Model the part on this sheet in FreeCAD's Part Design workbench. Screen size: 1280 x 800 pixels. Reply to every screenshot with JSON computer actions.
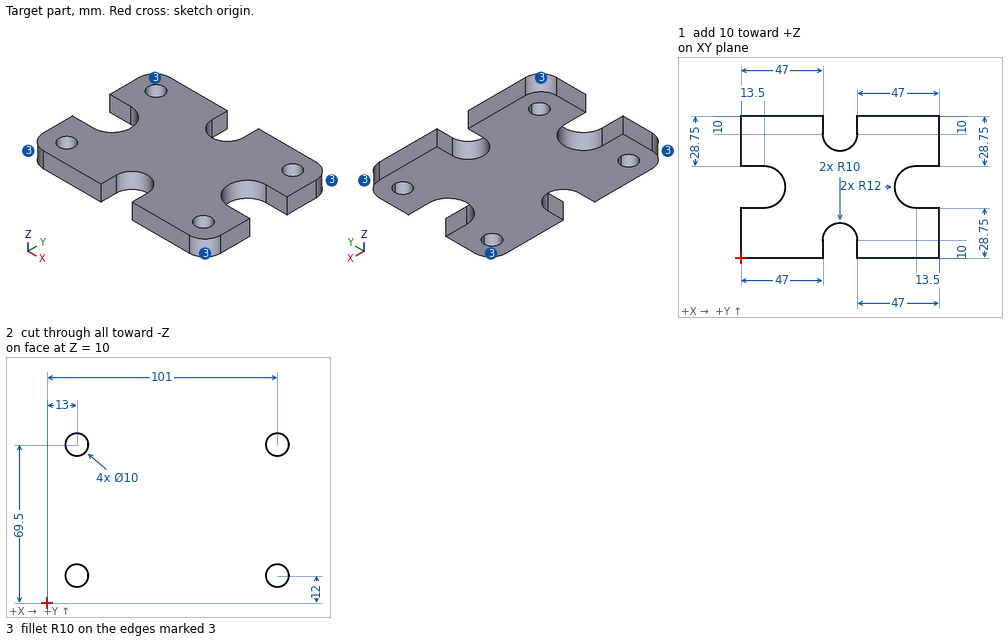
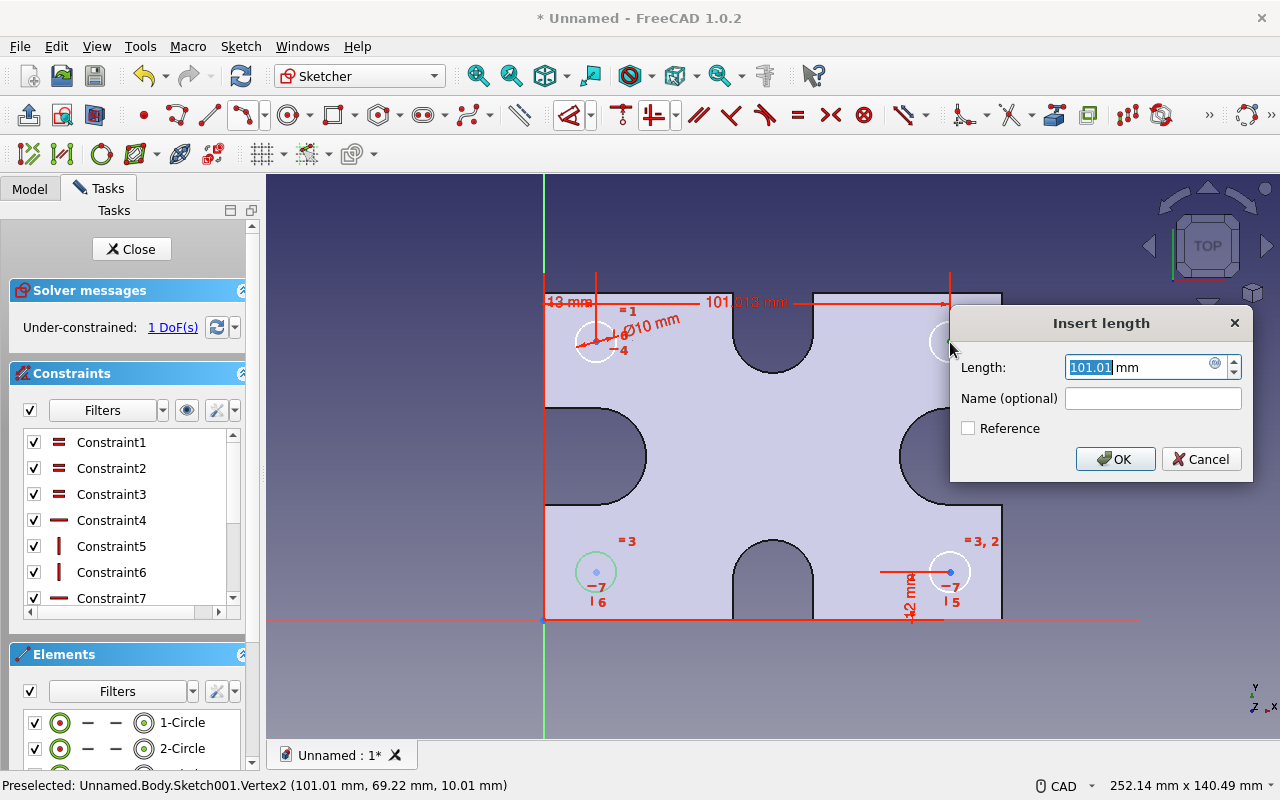
{"action": "type", "text": "101"}
{"action": "key", "text": "Return"}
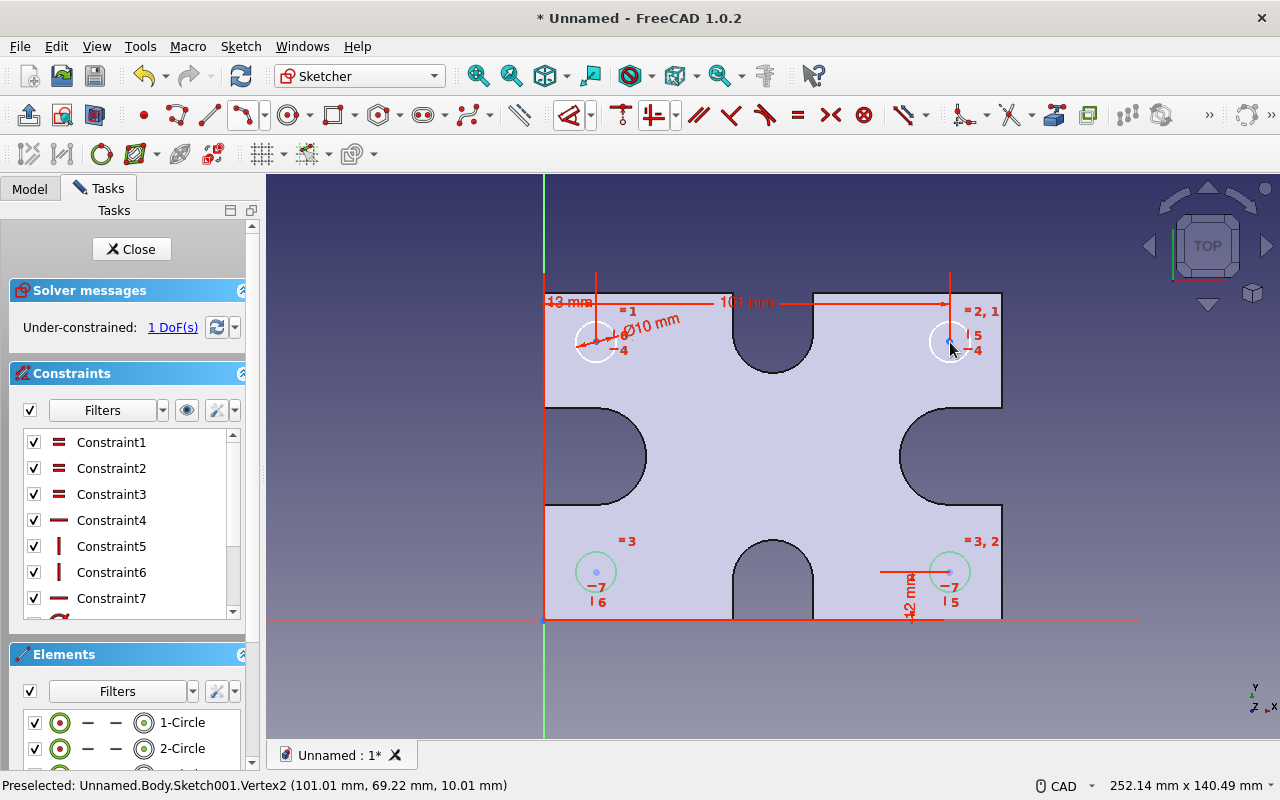
{"action": "left_click", "coordinate": [596, 342]}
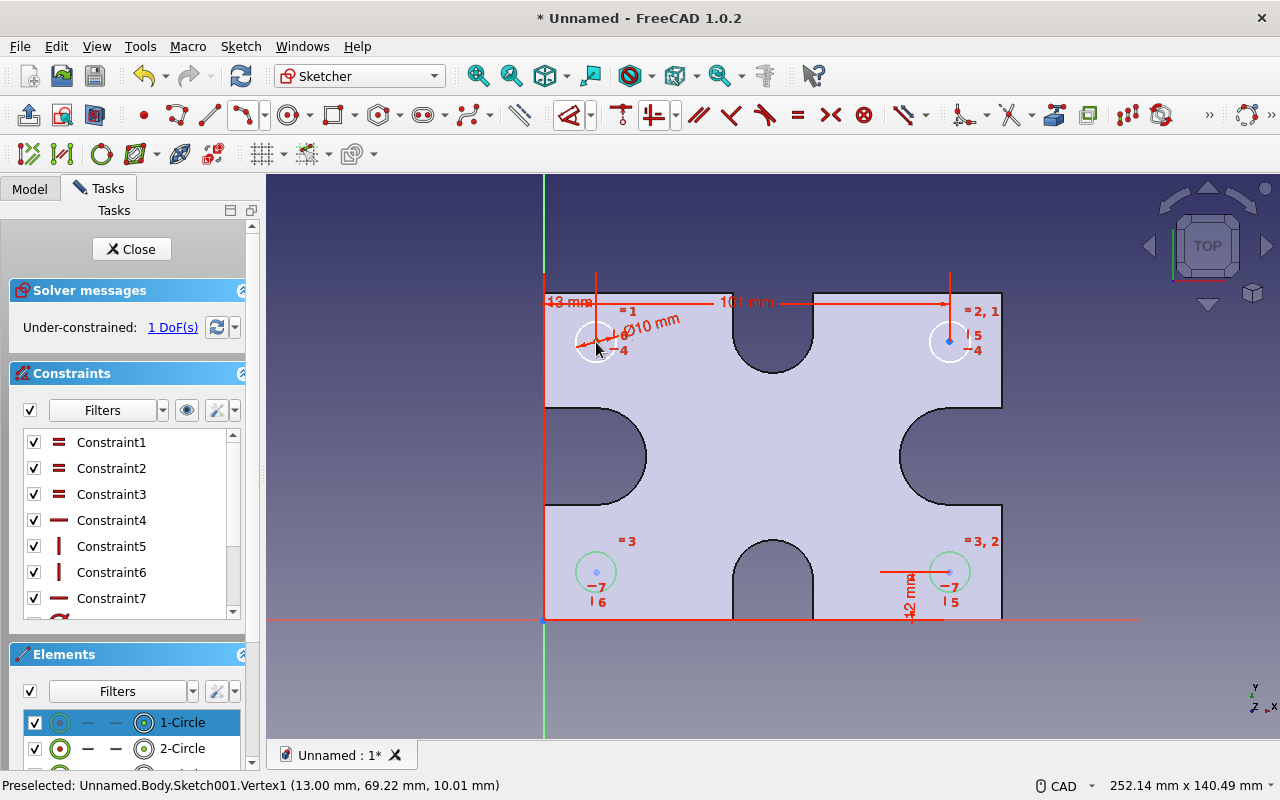
{"action": "left_click", "coordinate": [590, 116]}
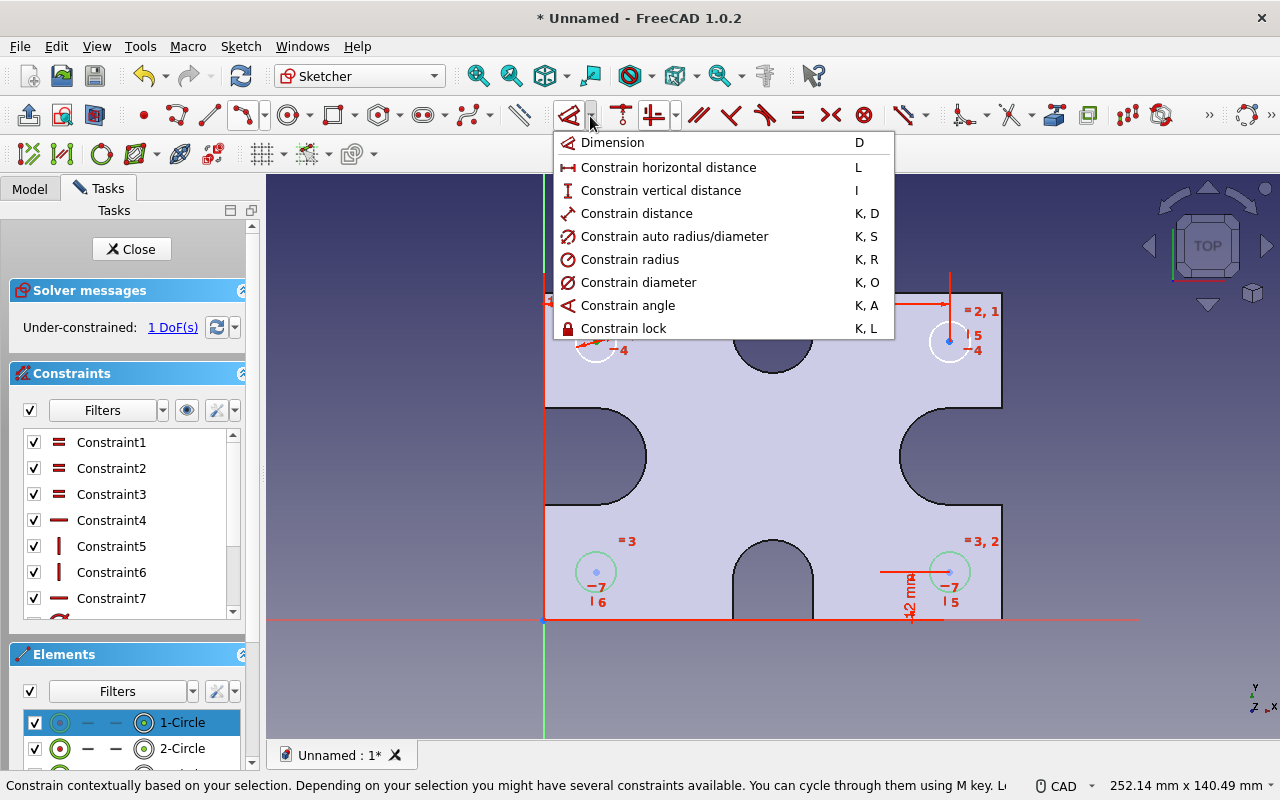
{"action": "left_click", "coordinate": [724, 190]}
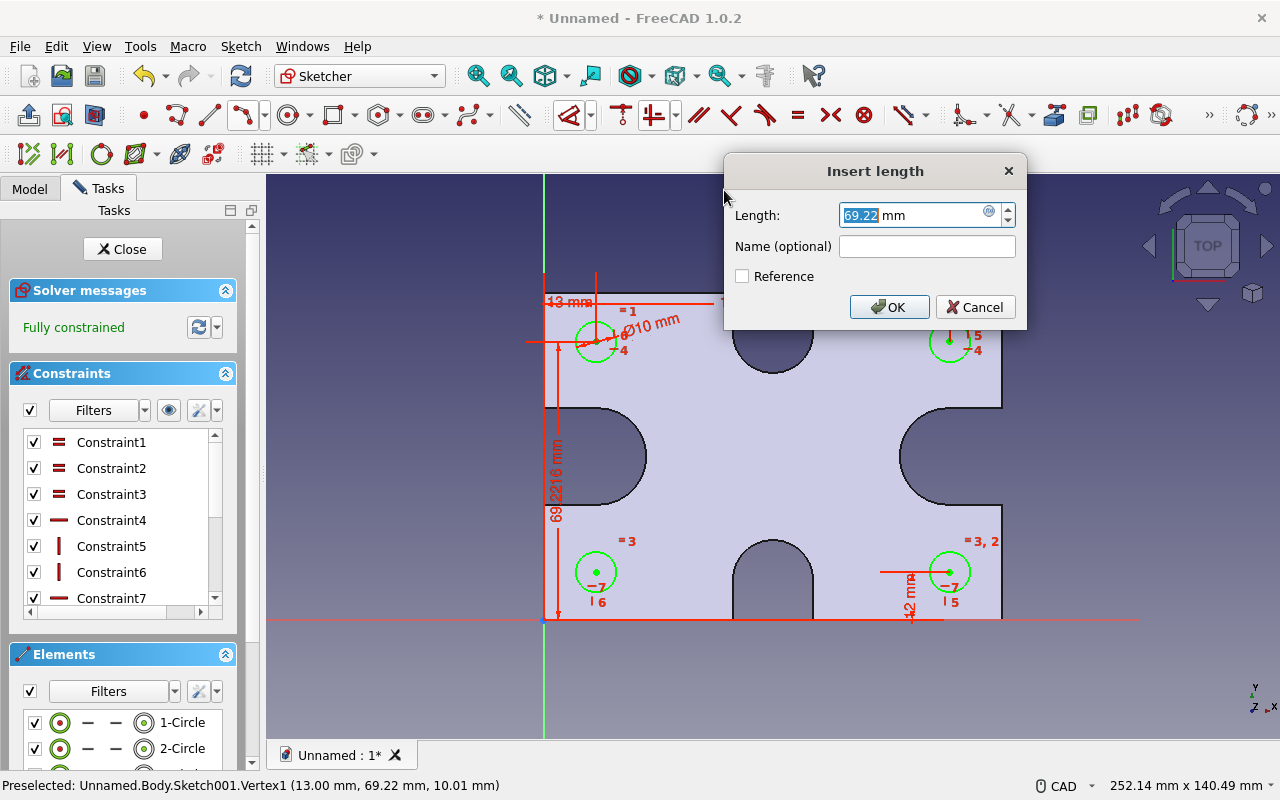
{"action": "type", "text": "69.5"}
{"action": "key", "text": "Return"}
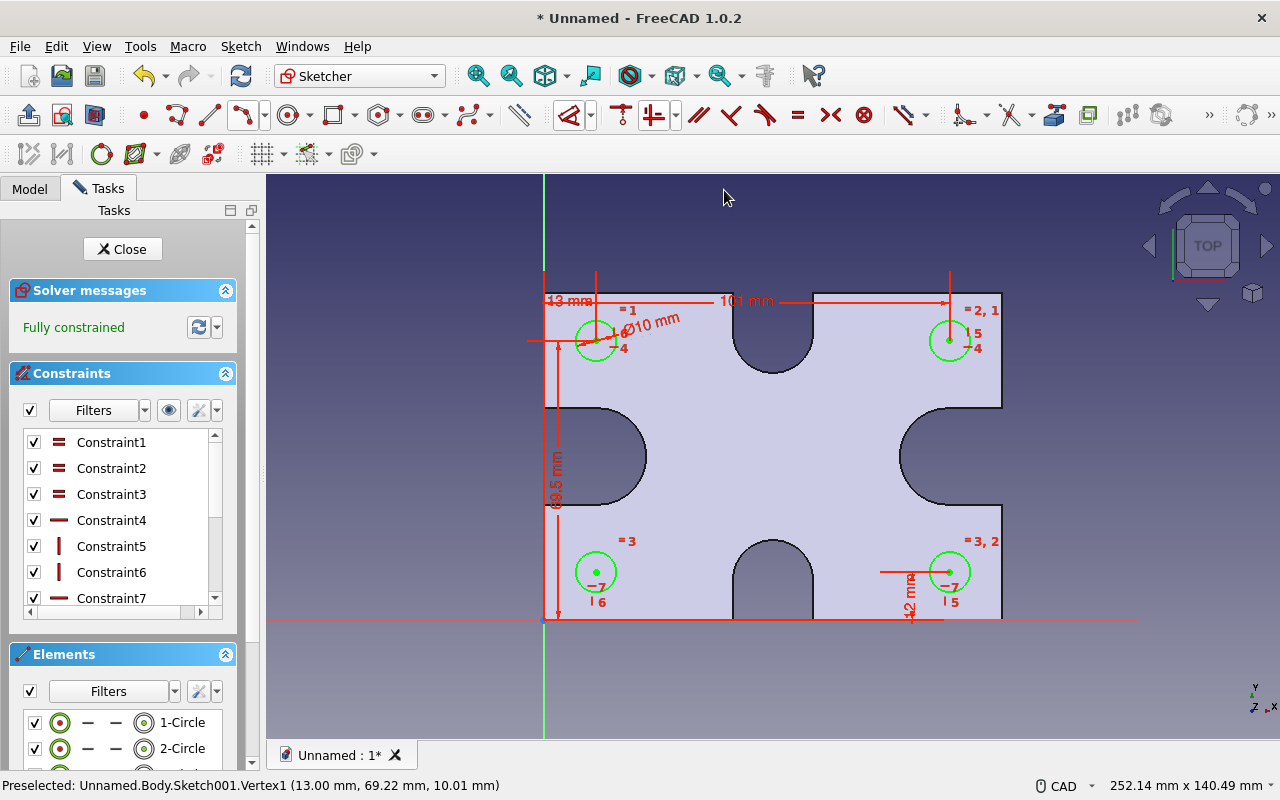
{"action": "left_click", "coordinate": [123, 249]}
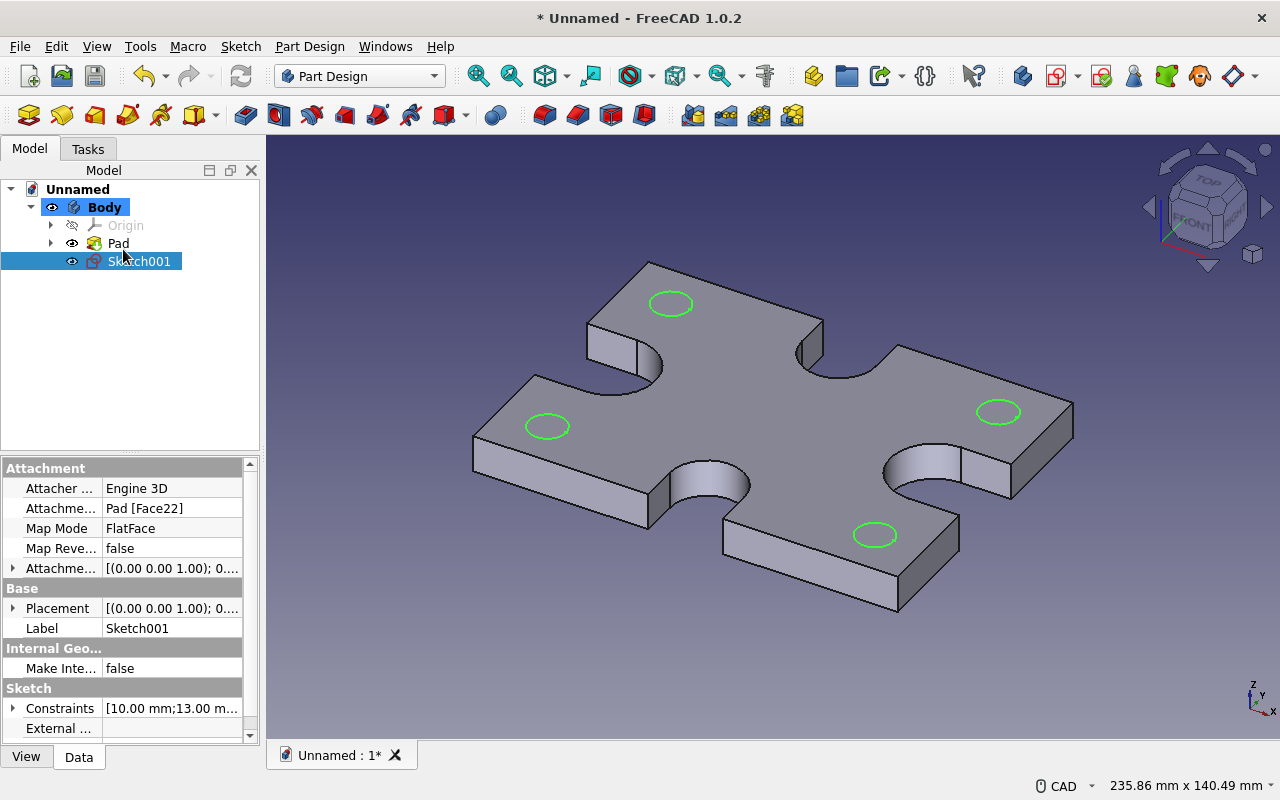
{"action": "left_click", "coordinate": [246, 116]}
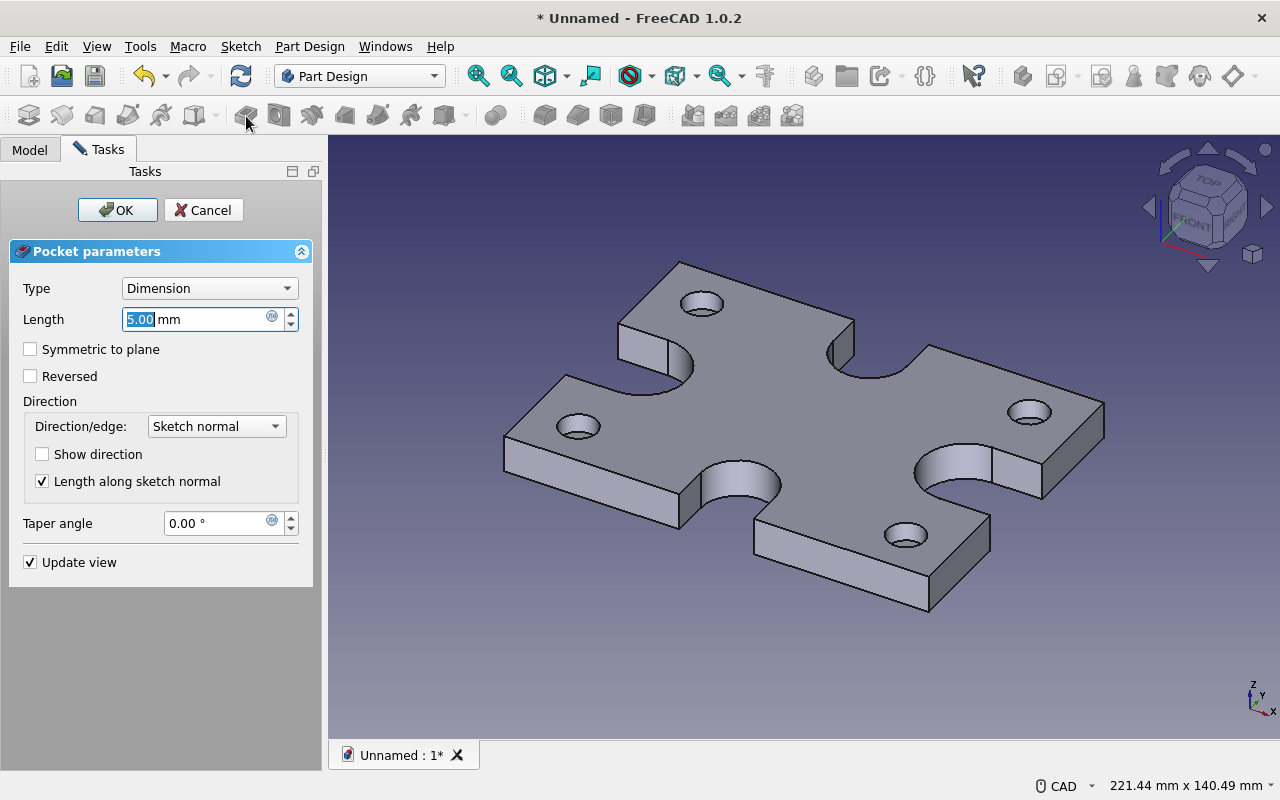
{"action": "left_click", "coordinate": [210, 288]}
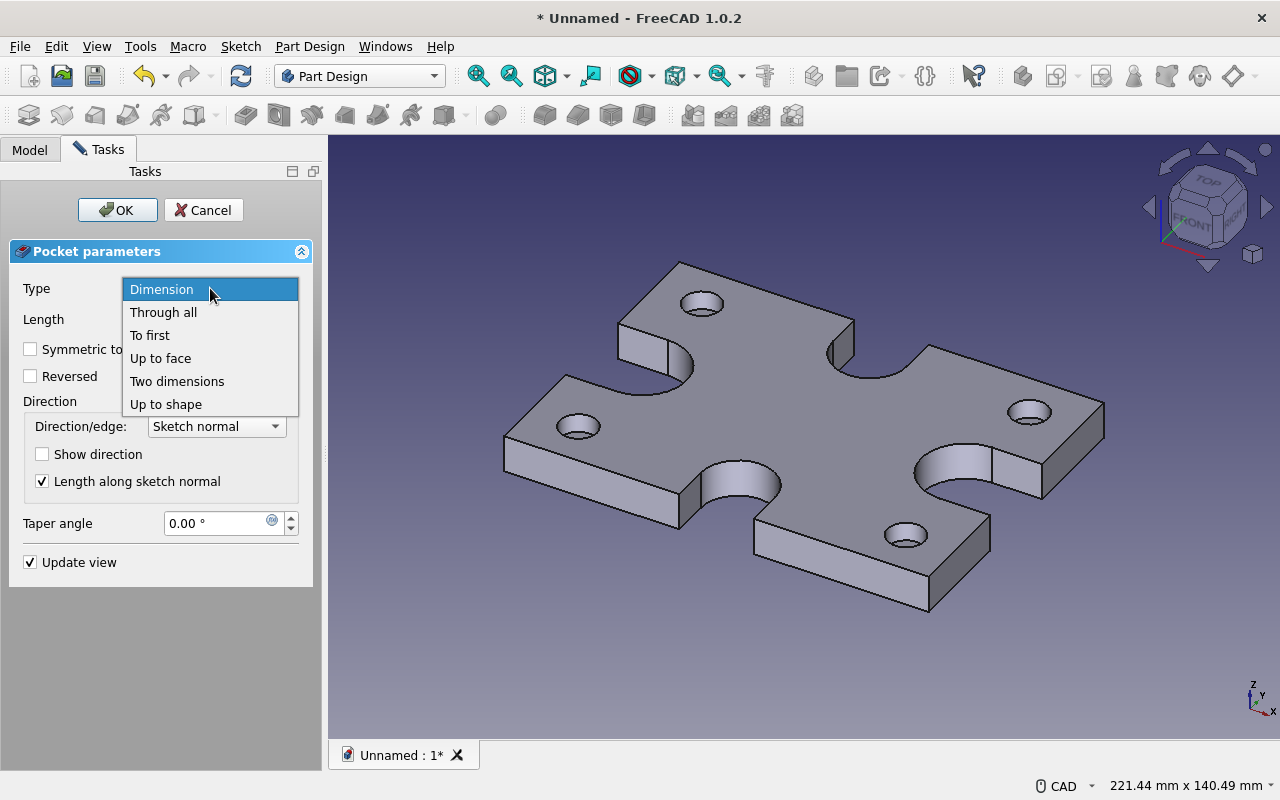
{"action": "left_click", "coordinate": [208, 312]}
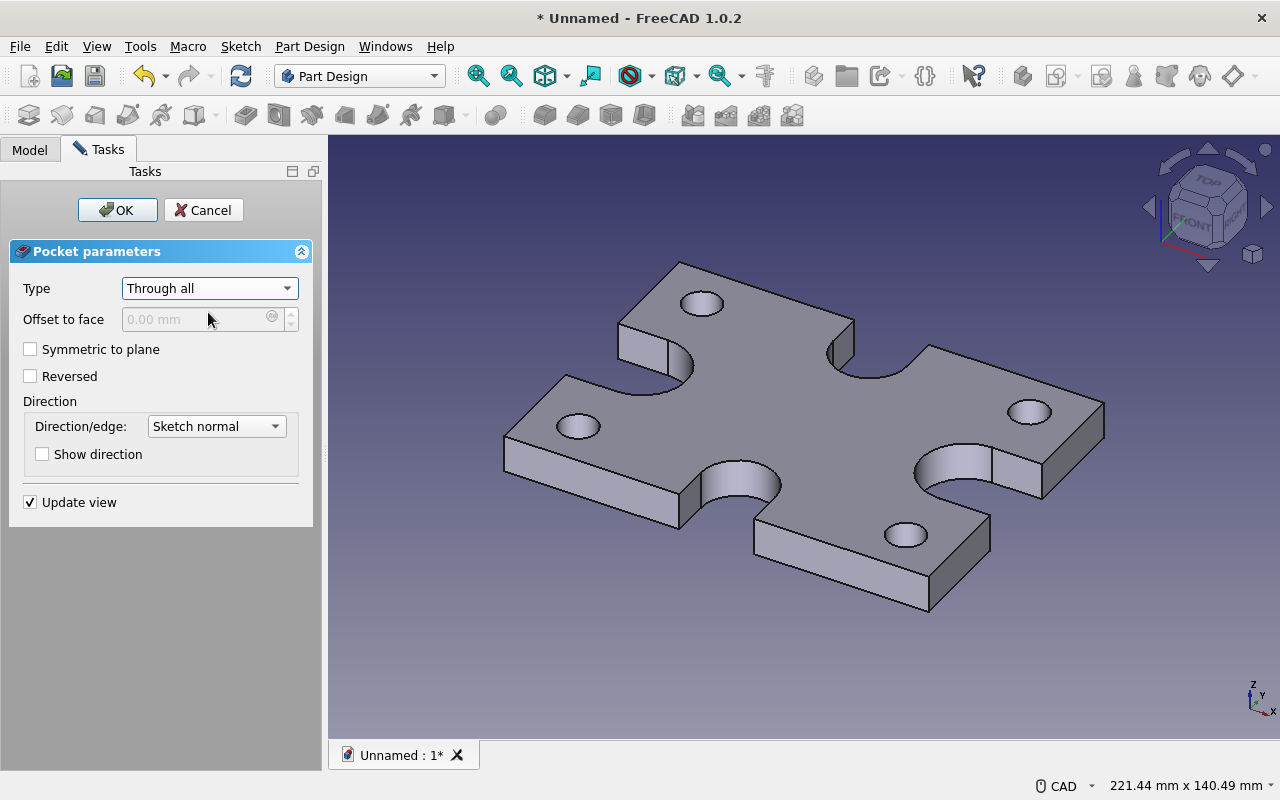
{"action": "left_click", "coordinate": [118, 210]}